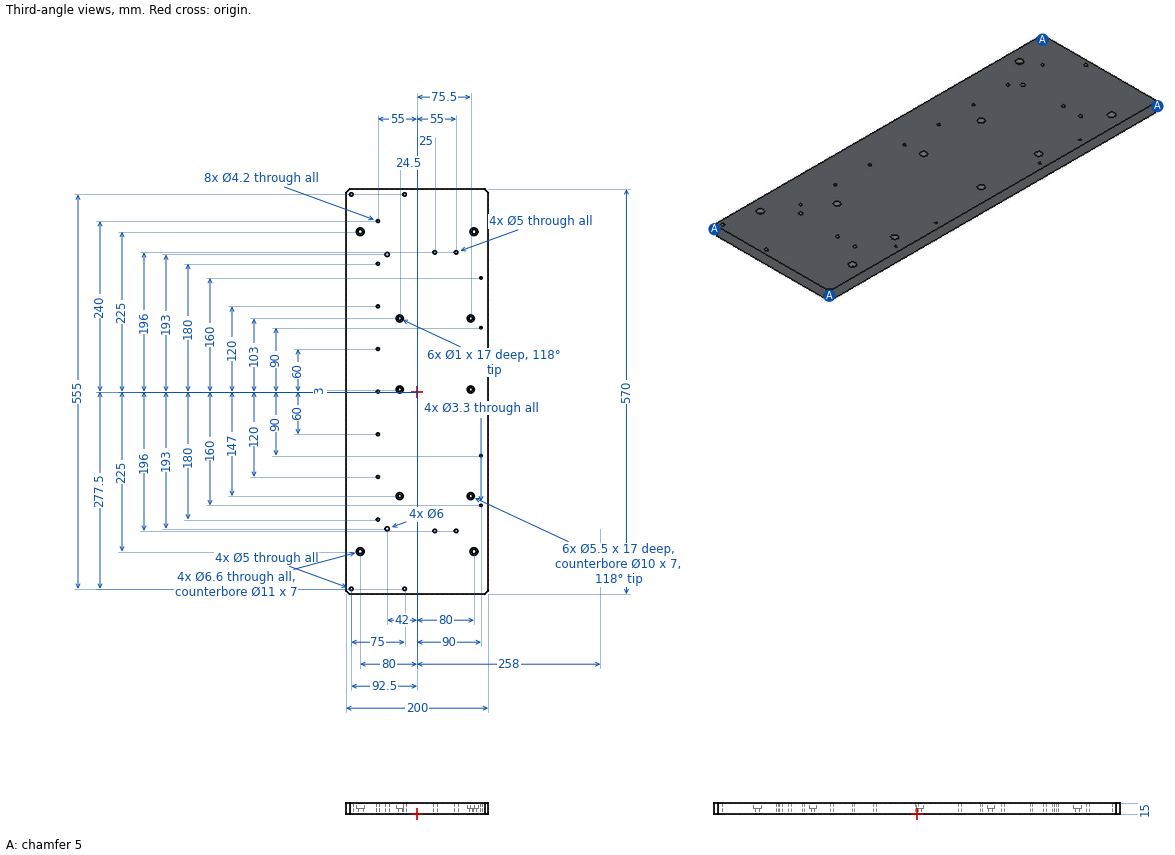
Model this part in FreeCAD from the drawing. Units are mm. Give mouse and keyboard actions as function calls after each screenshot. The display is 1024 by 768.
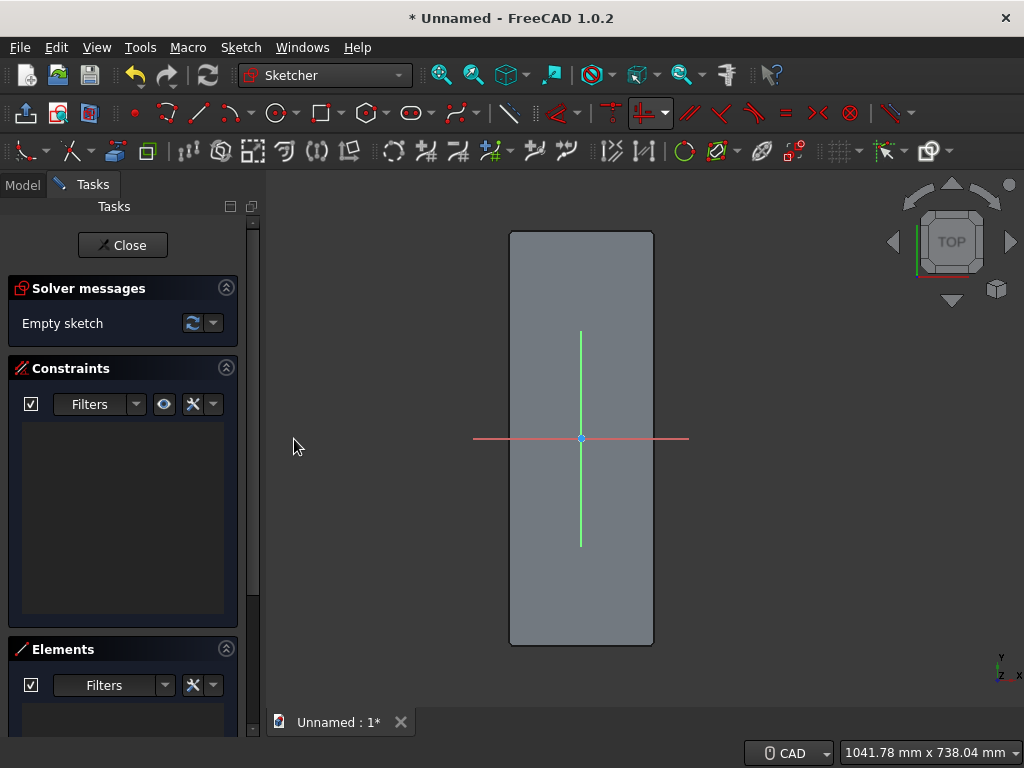
click(276, 114)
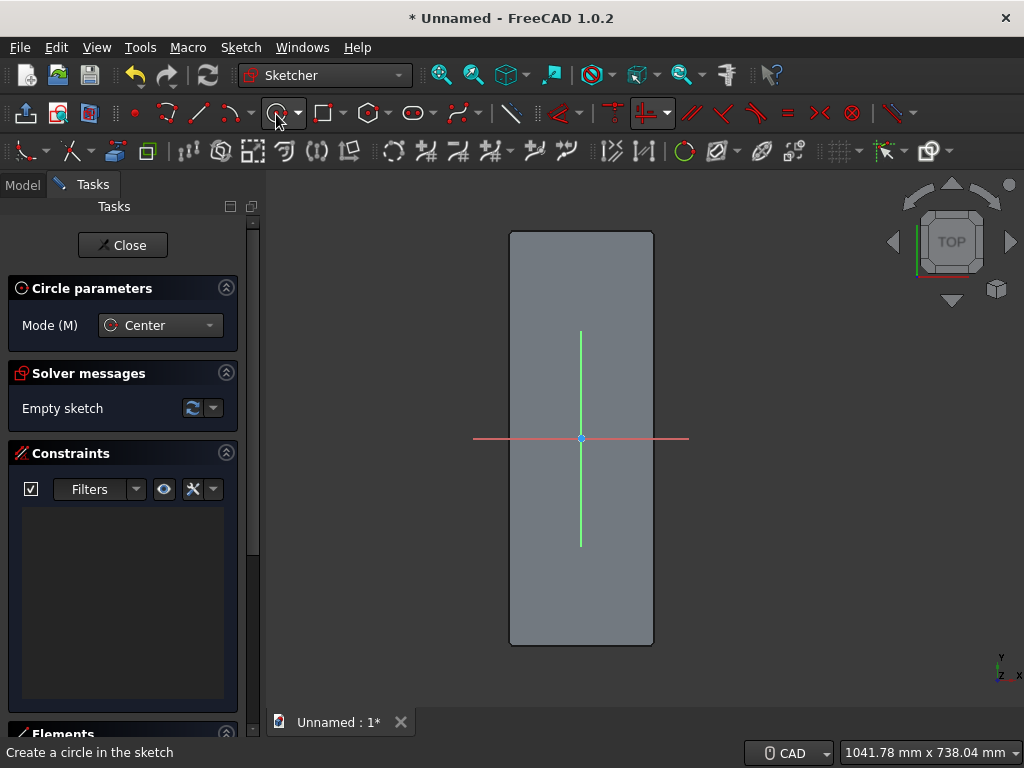
scroll(551, 579, up, 12)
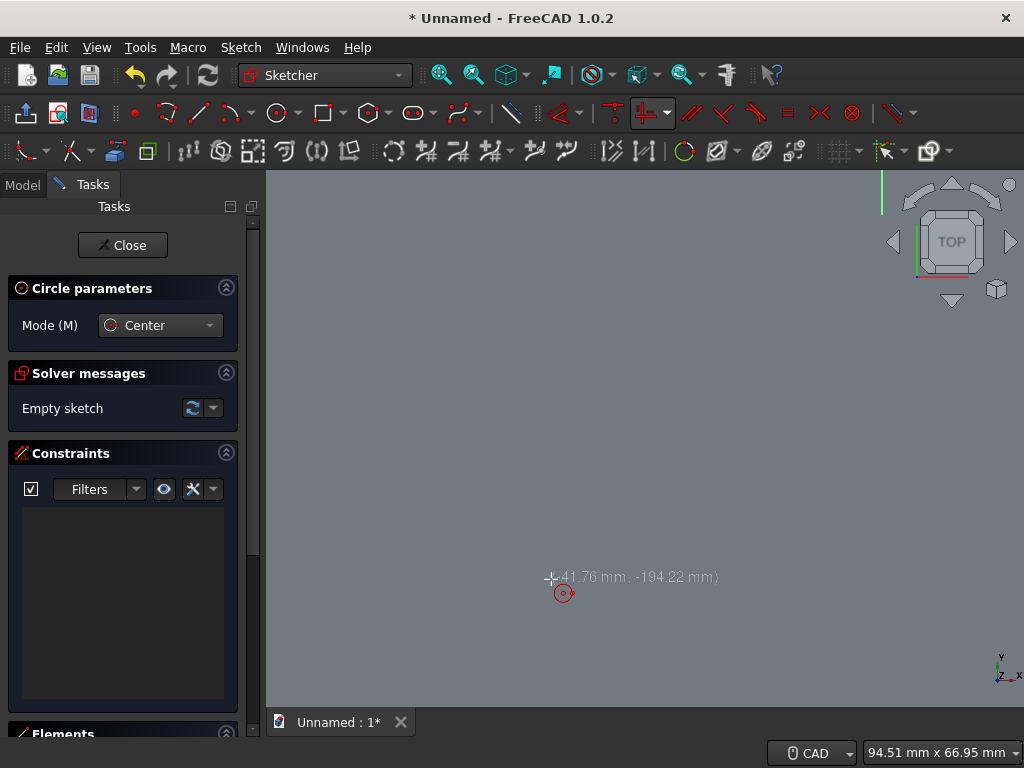
scroll(430, 615, down, 11)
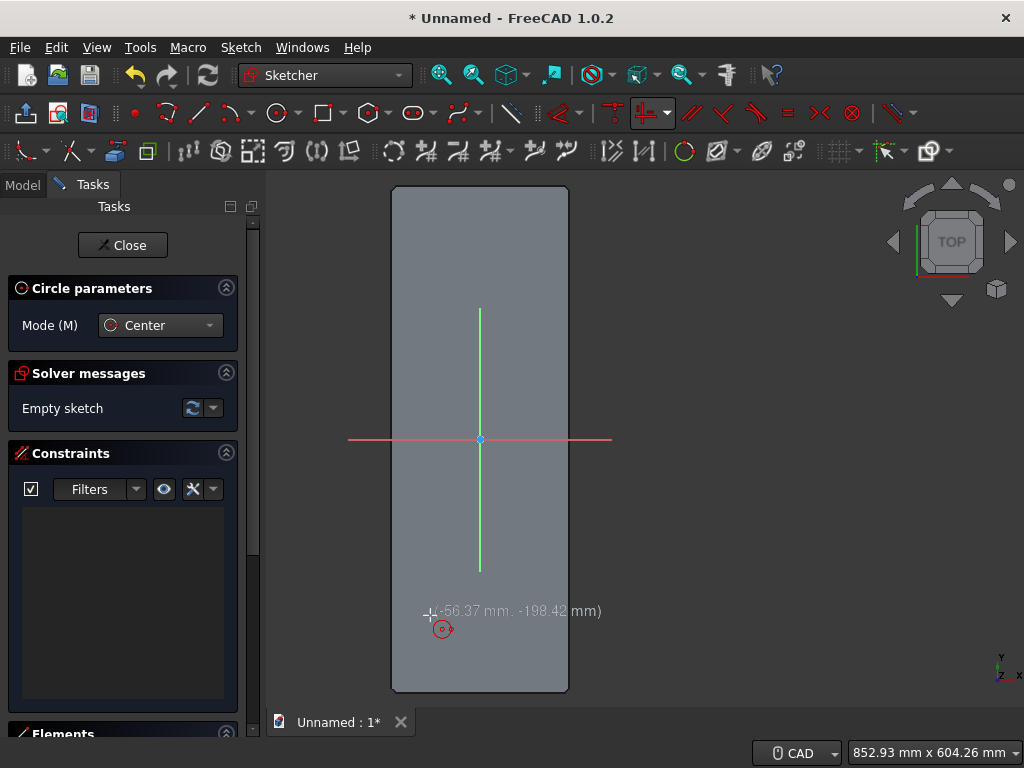
click(443, 611)
move(445, 609)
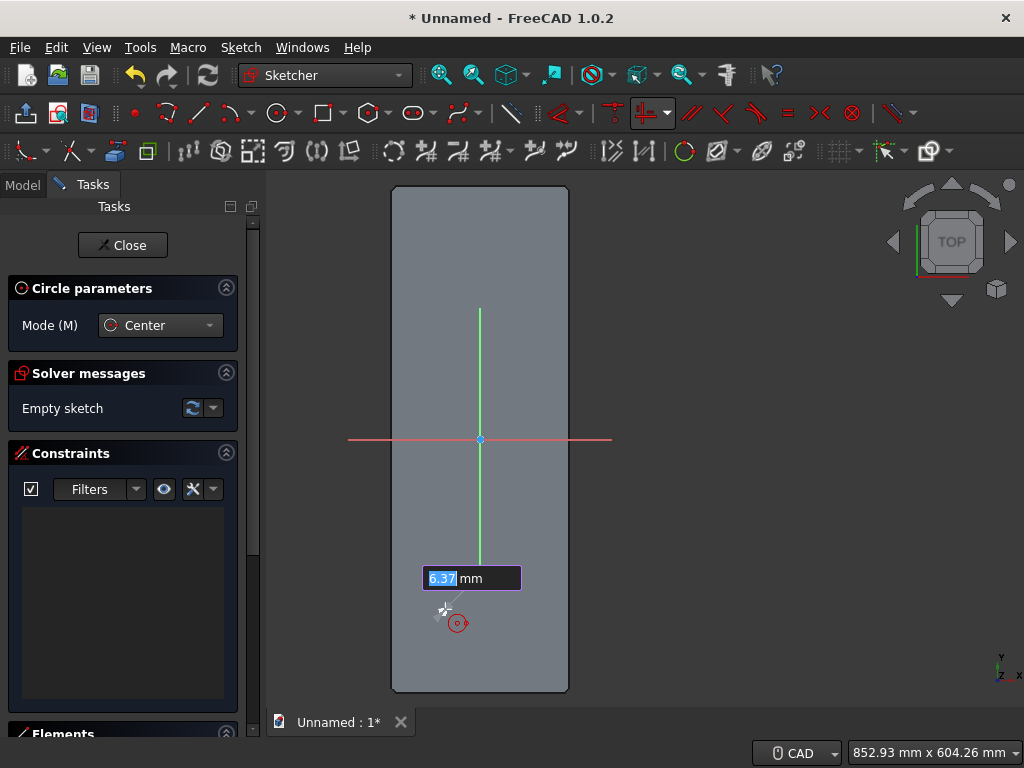
text(6)
key(Return)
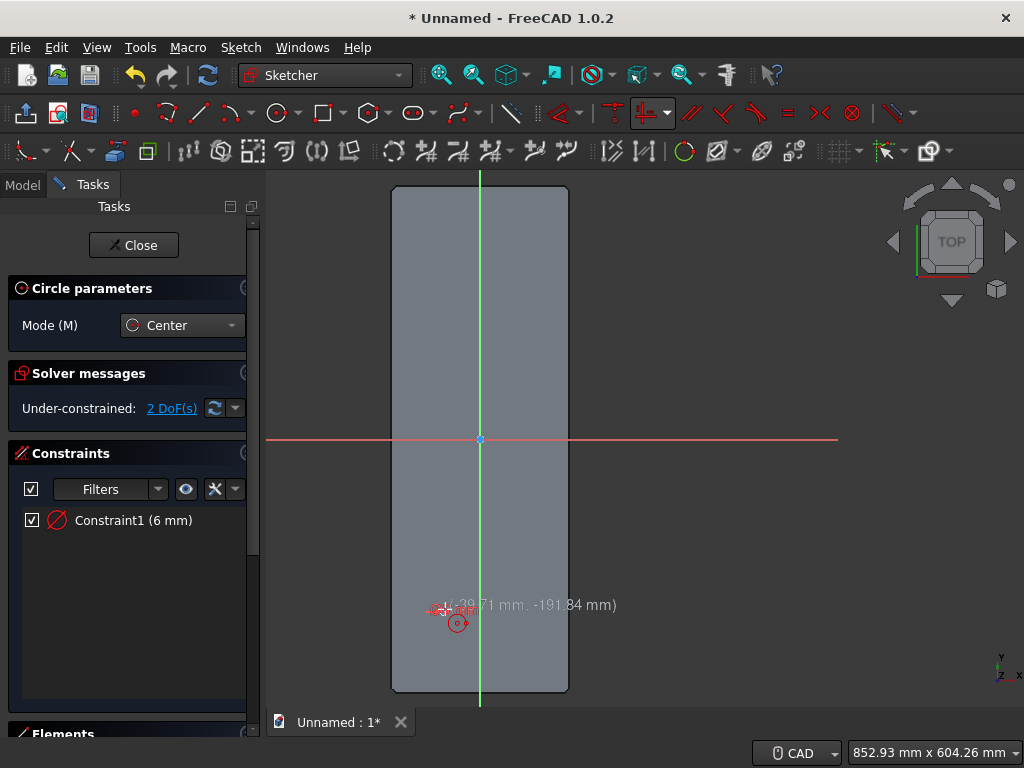
scroll(710, 611, up, 11)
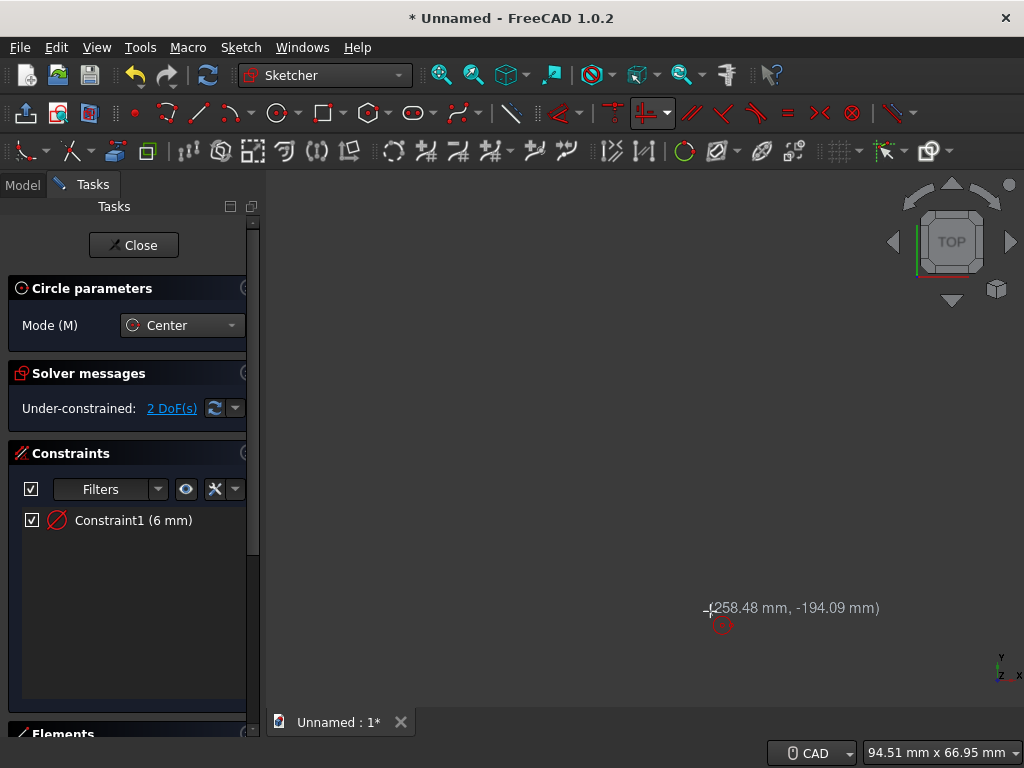
scroll(711, 611, down, 11)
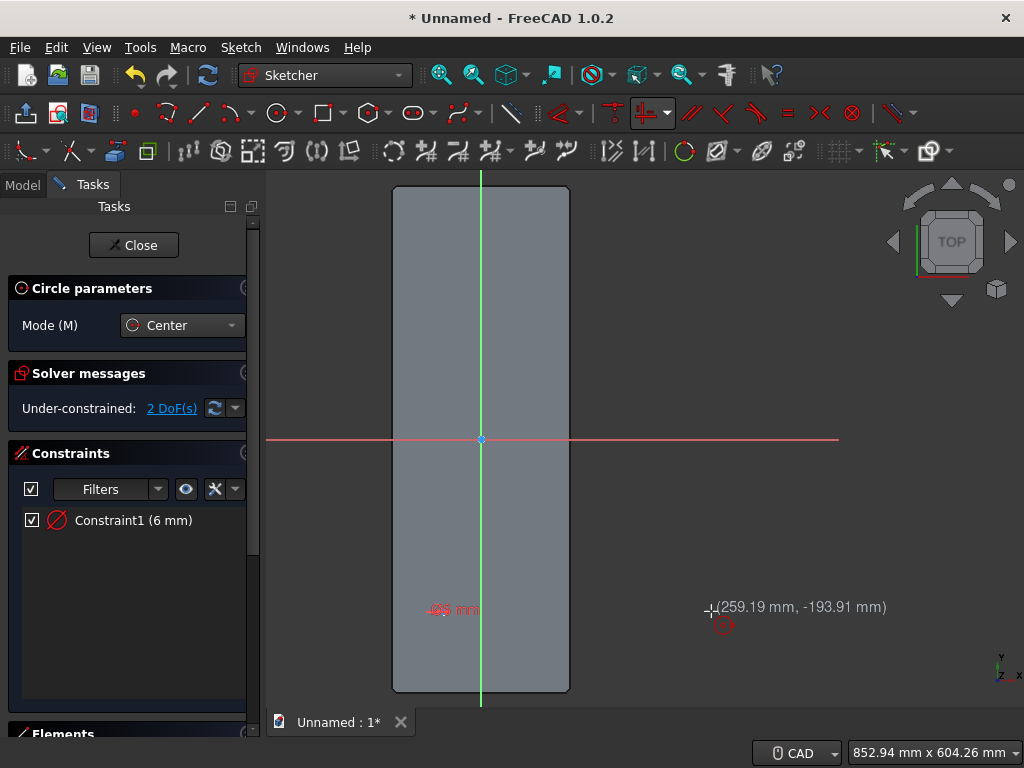
click(710, 611)
move(712, 609)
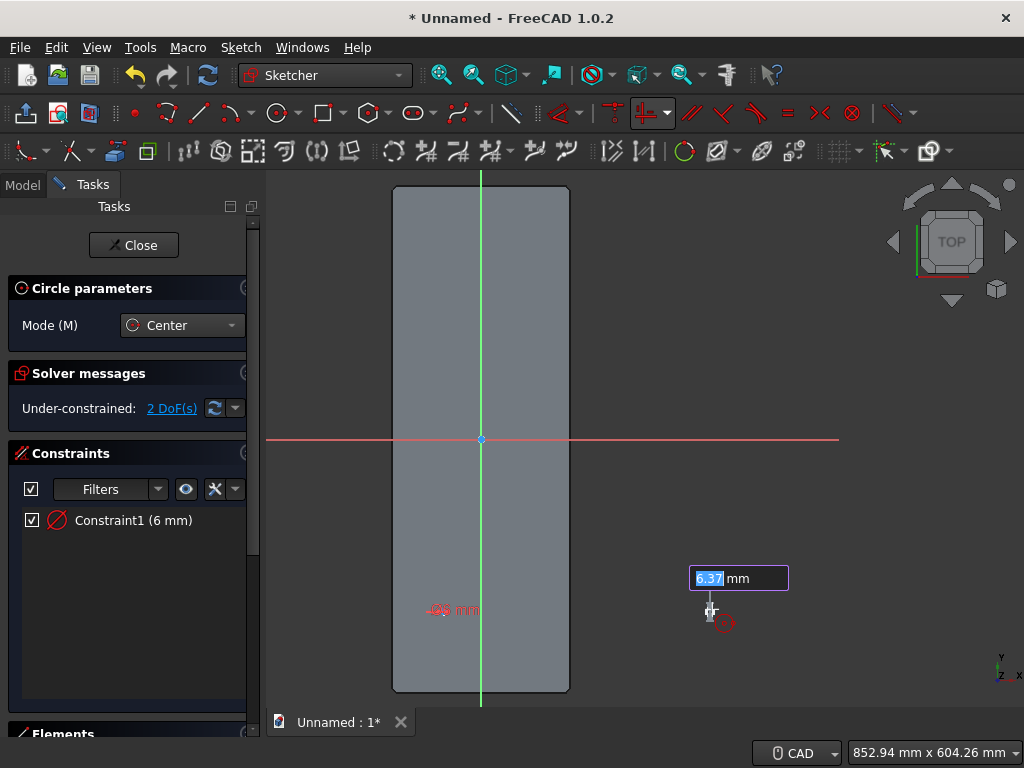
text(6)
key(Return)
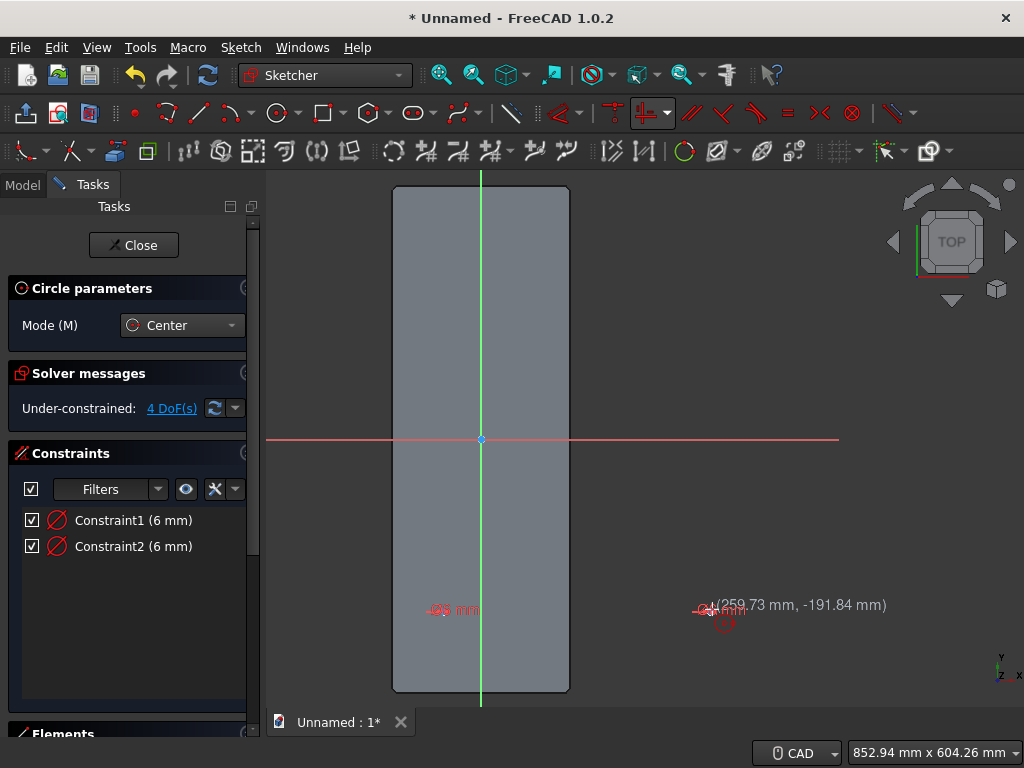
scroll(444, 268, up, 11)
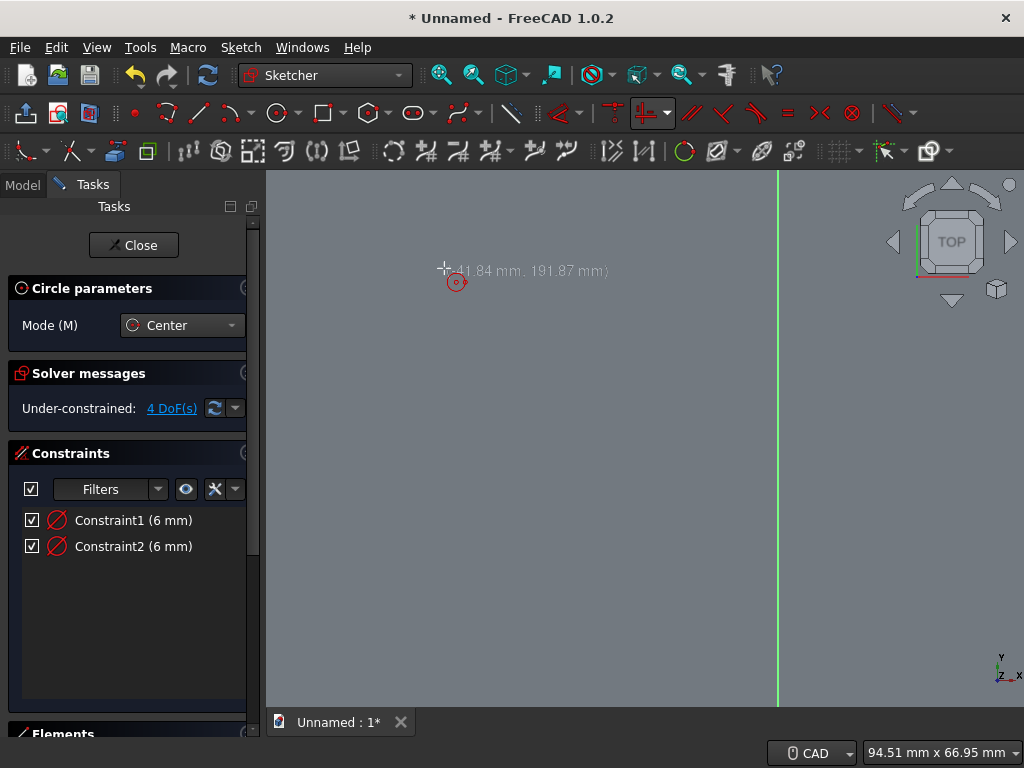
scroll(443, 267, down, 11)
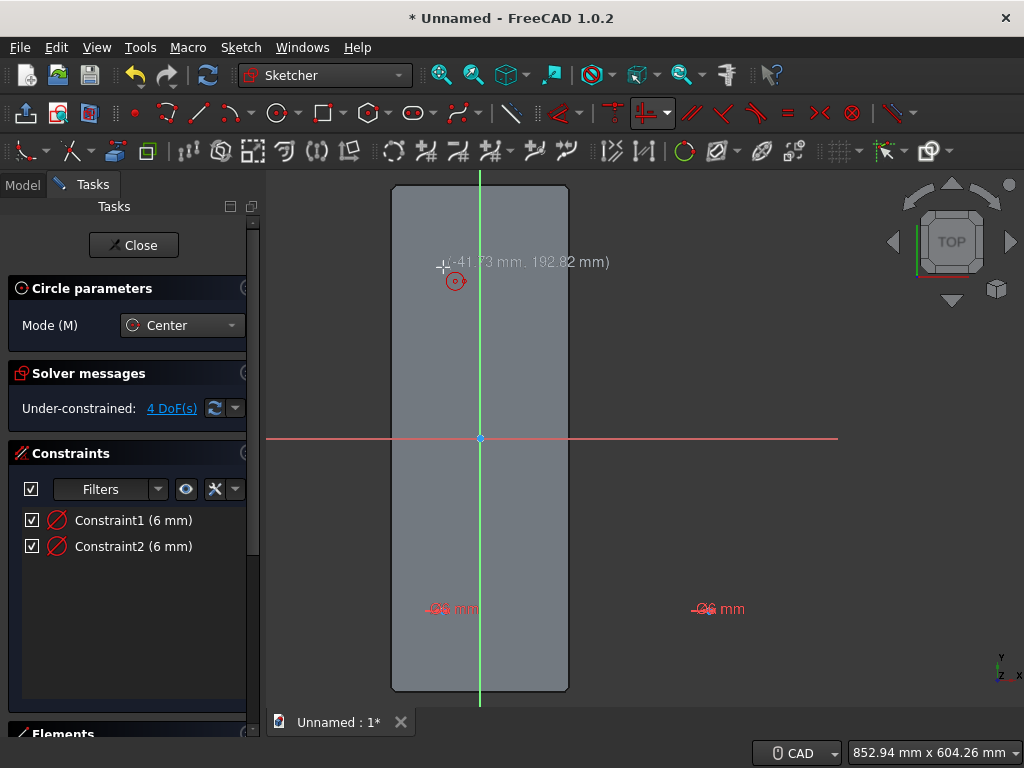
click(443, 267)
move(445, 265)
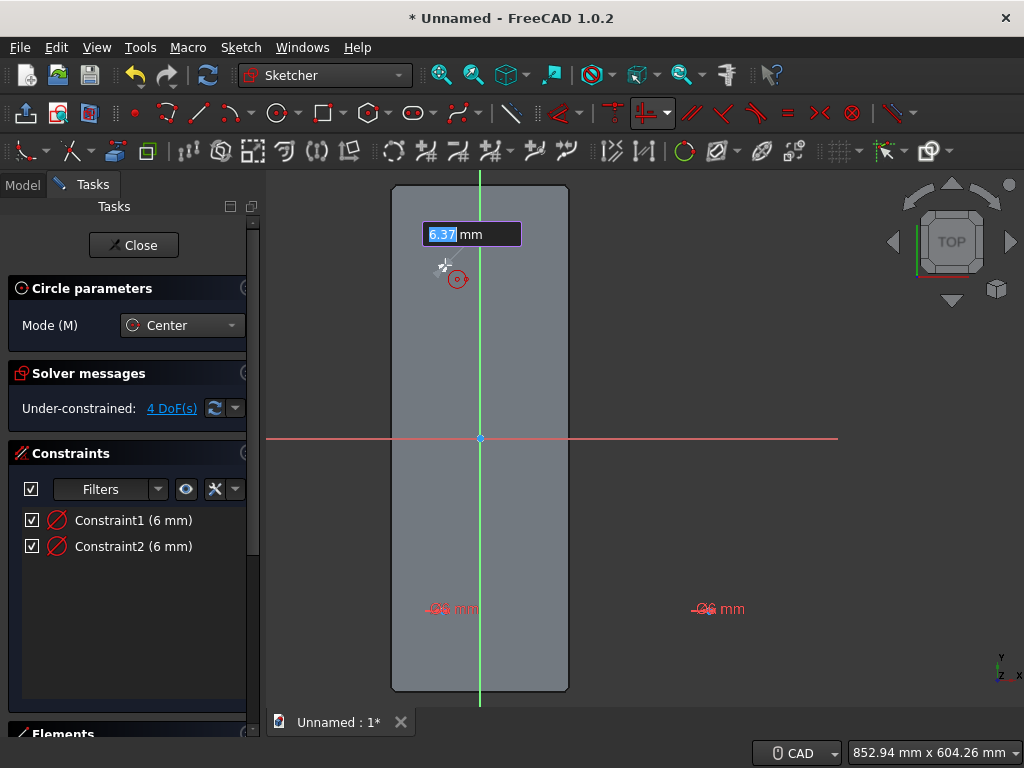
text(6)
key(Return)